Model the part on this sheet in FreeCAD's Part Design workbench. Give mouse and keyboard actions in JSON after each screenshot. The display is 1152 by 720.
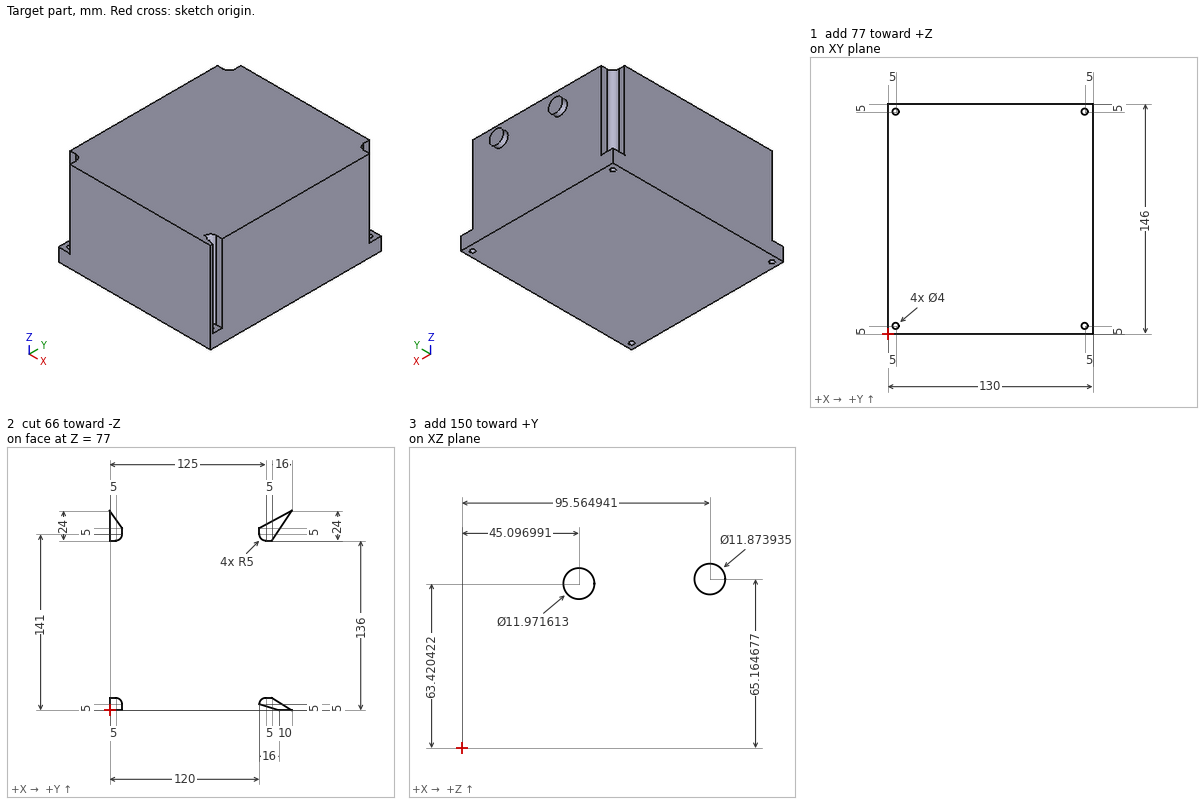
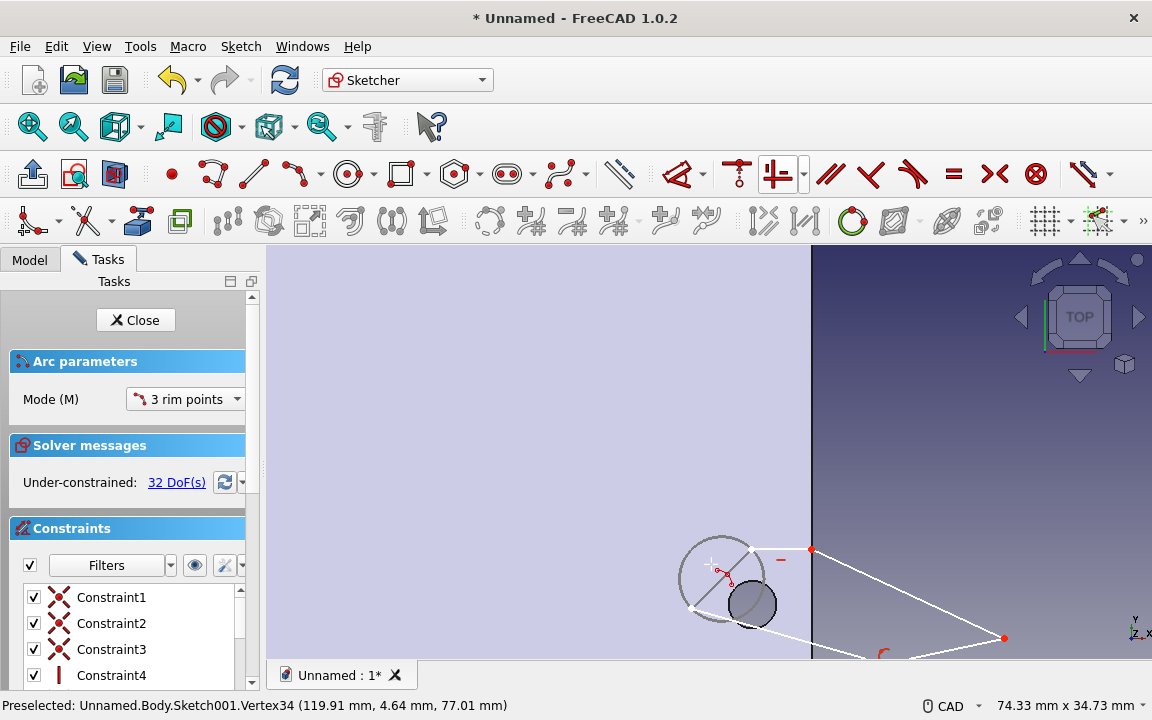
{"action": "left_click", "coordinate": [710, 562]}
{"action": "key", "text": "Escape"}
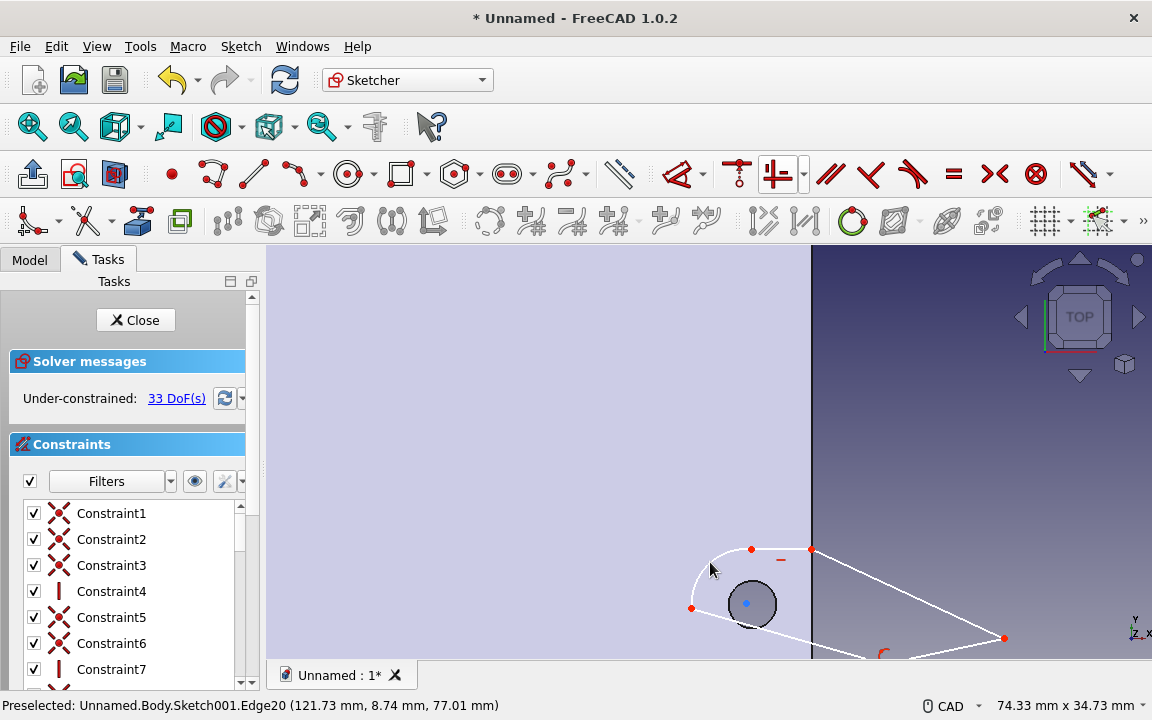
{"action": "scroll", "coordinate": [720, 568], "scroll_direction": "down", "scroll_amount": 10}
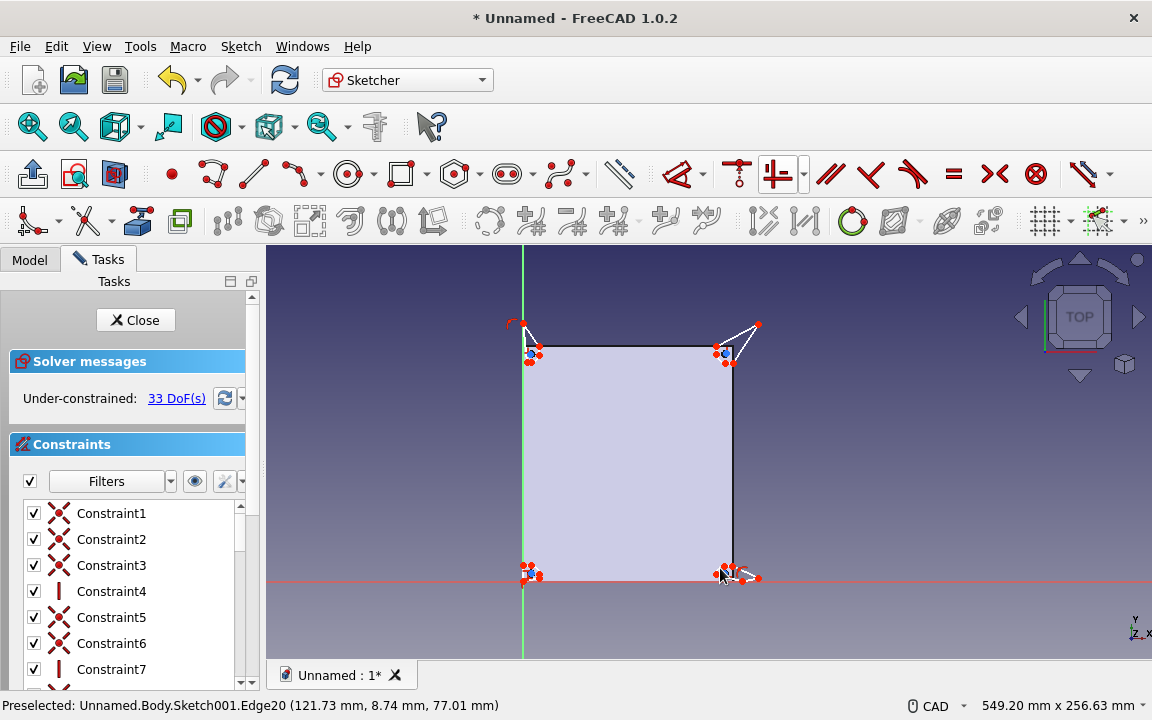
{"action": "scroll", "coordinate": [728, 363], "scroll_direction": "up", "scroll_amount": 9}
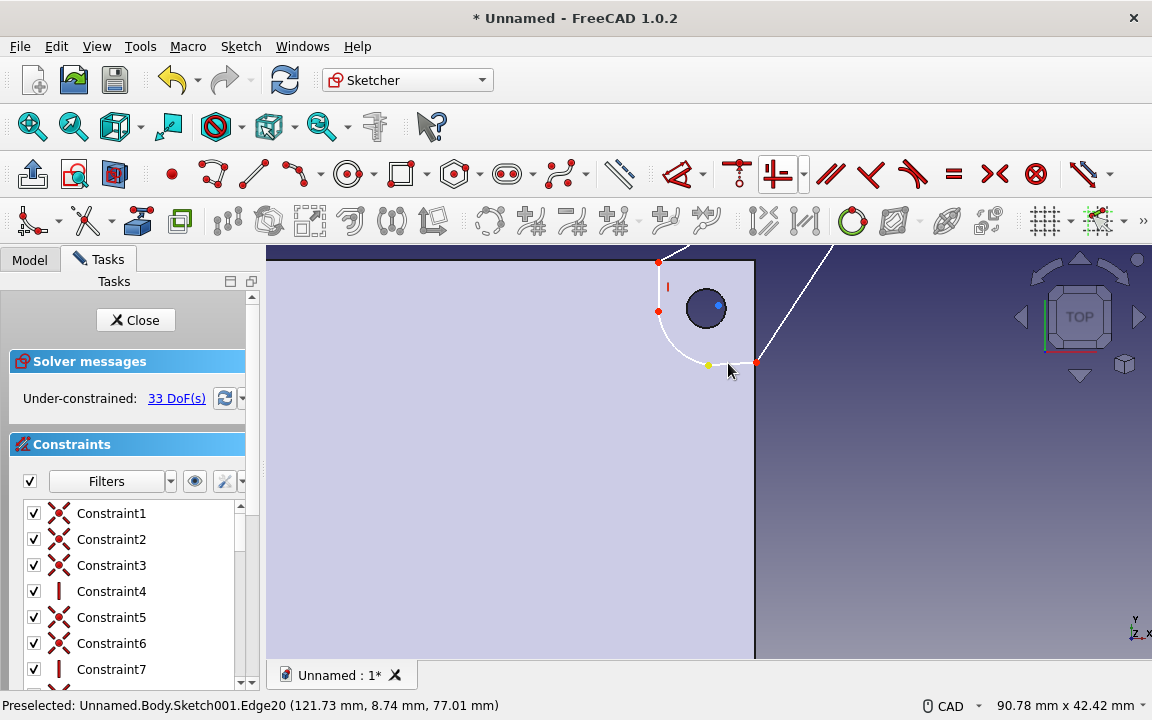
{"action": "left_click", "coordinate": [723, 364]}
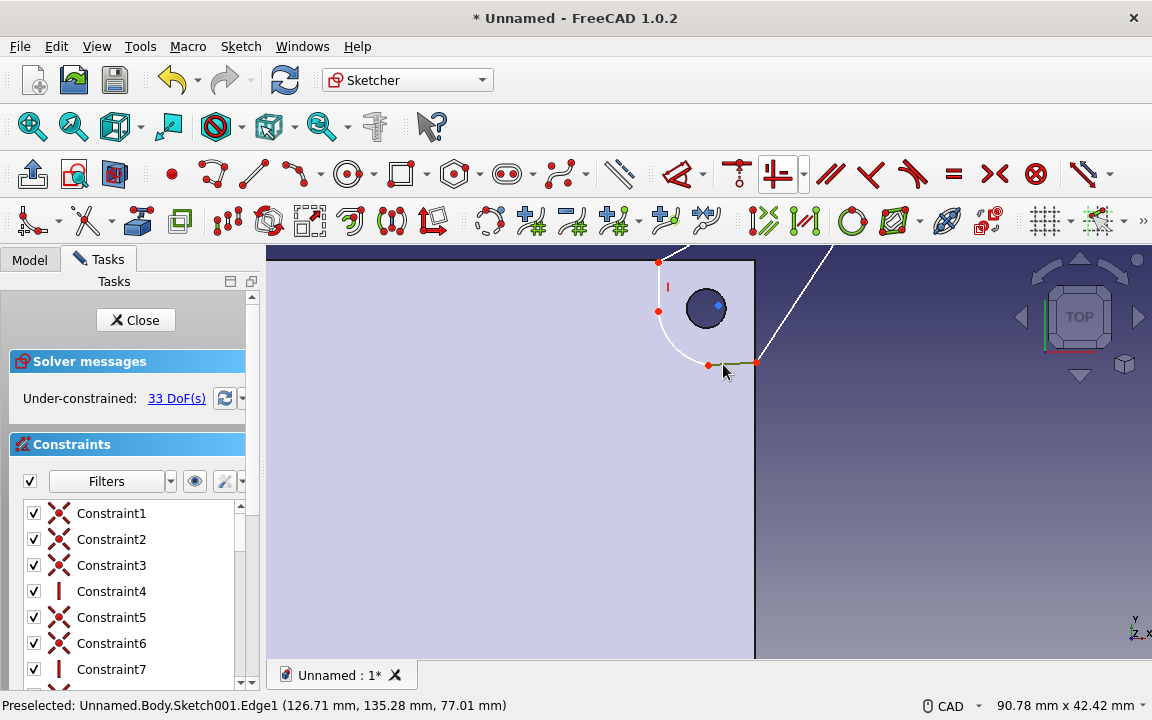
{"action": "left_click", "coordinate": [665, 334]}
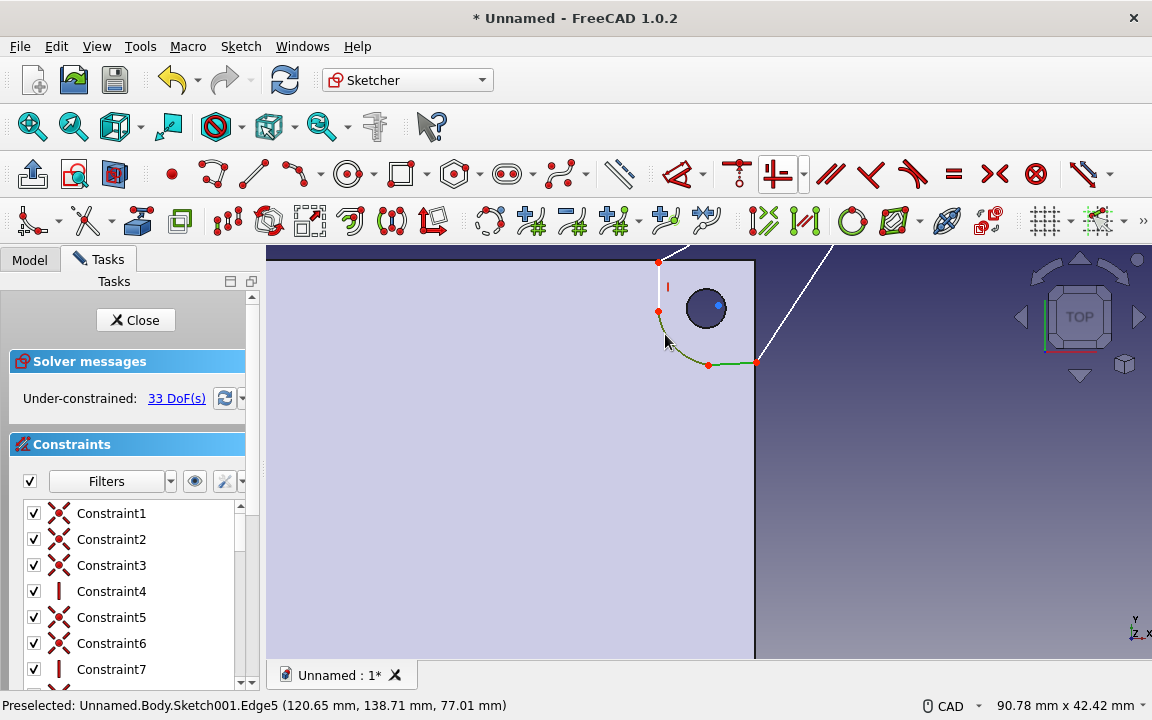
{"action": "left_click", "coordinate": [913, 174]}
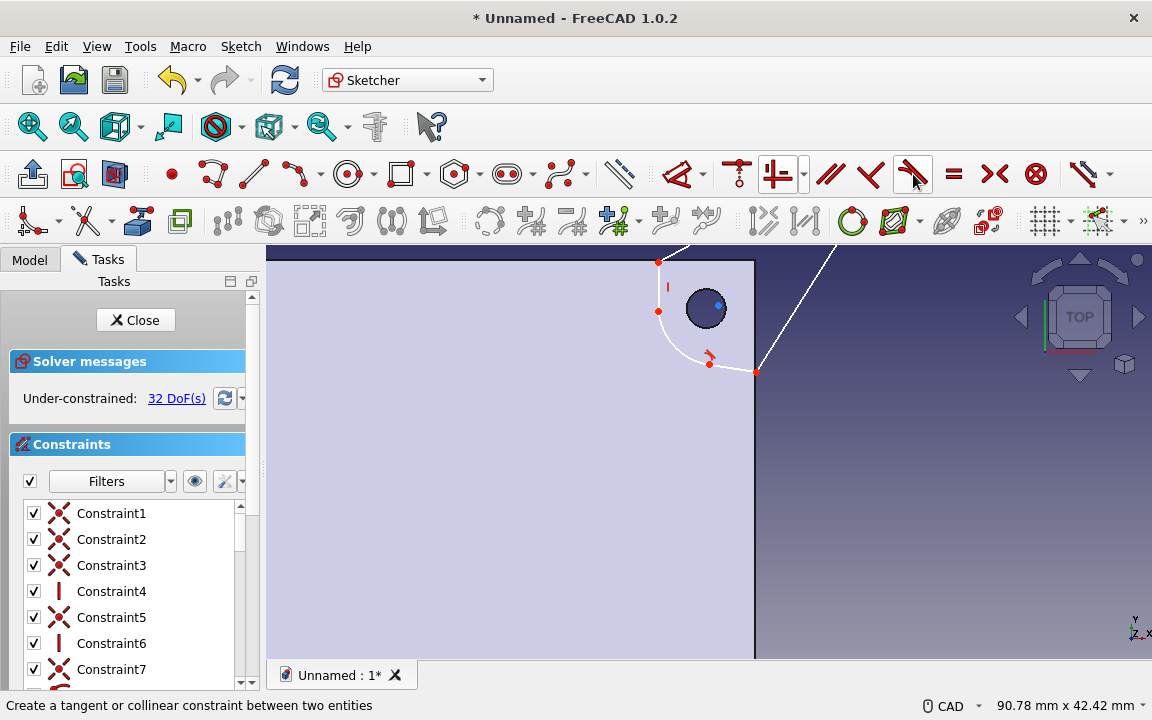
{"action": "left_click", "coordinate": [659, 277]}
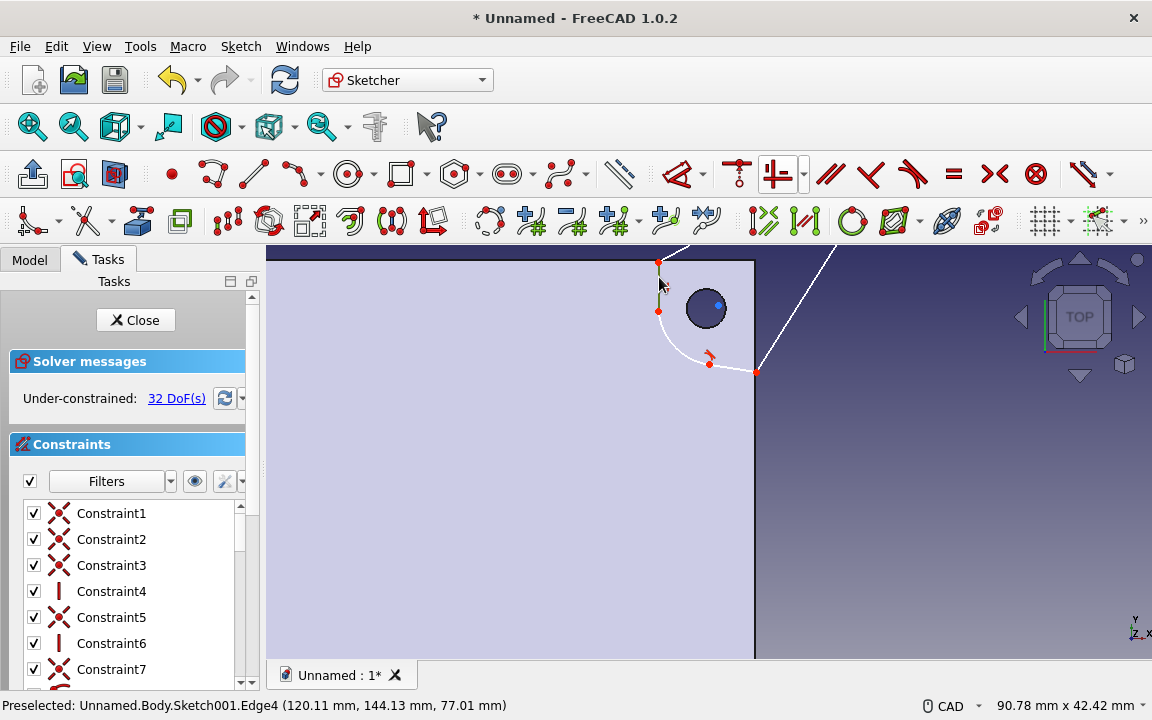
{"action": "left_click", "coordinate": [665, 334]}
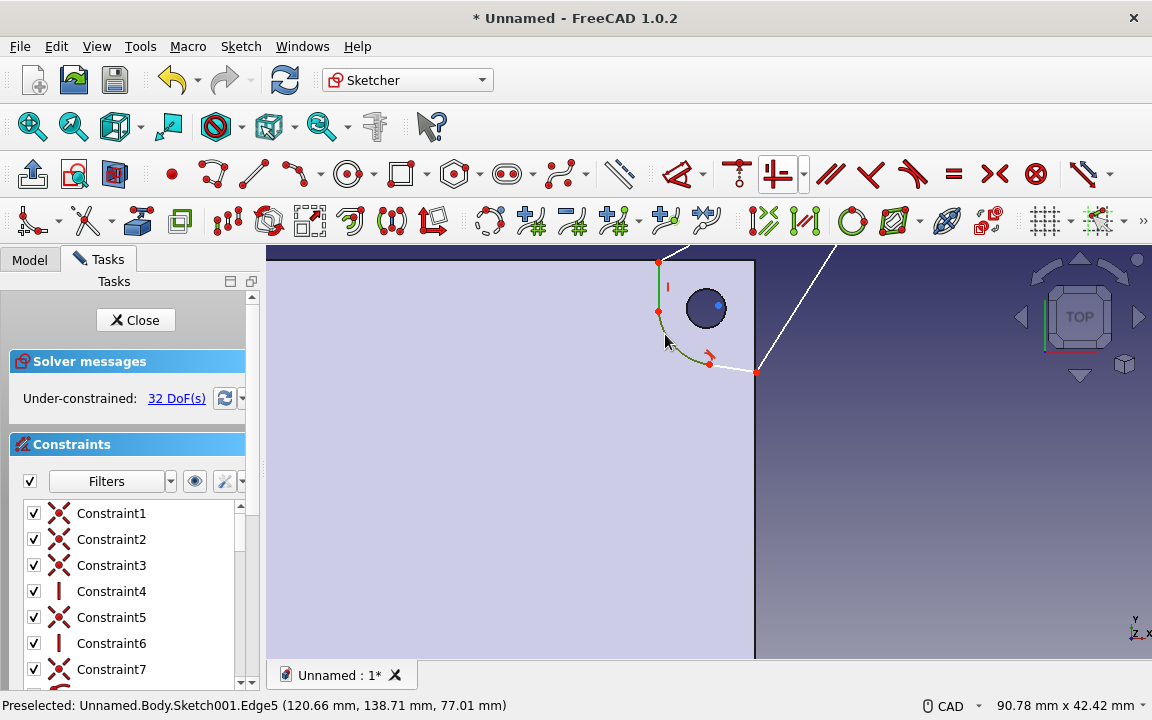
{"action": "left_click", "coordinate": [913, 174]}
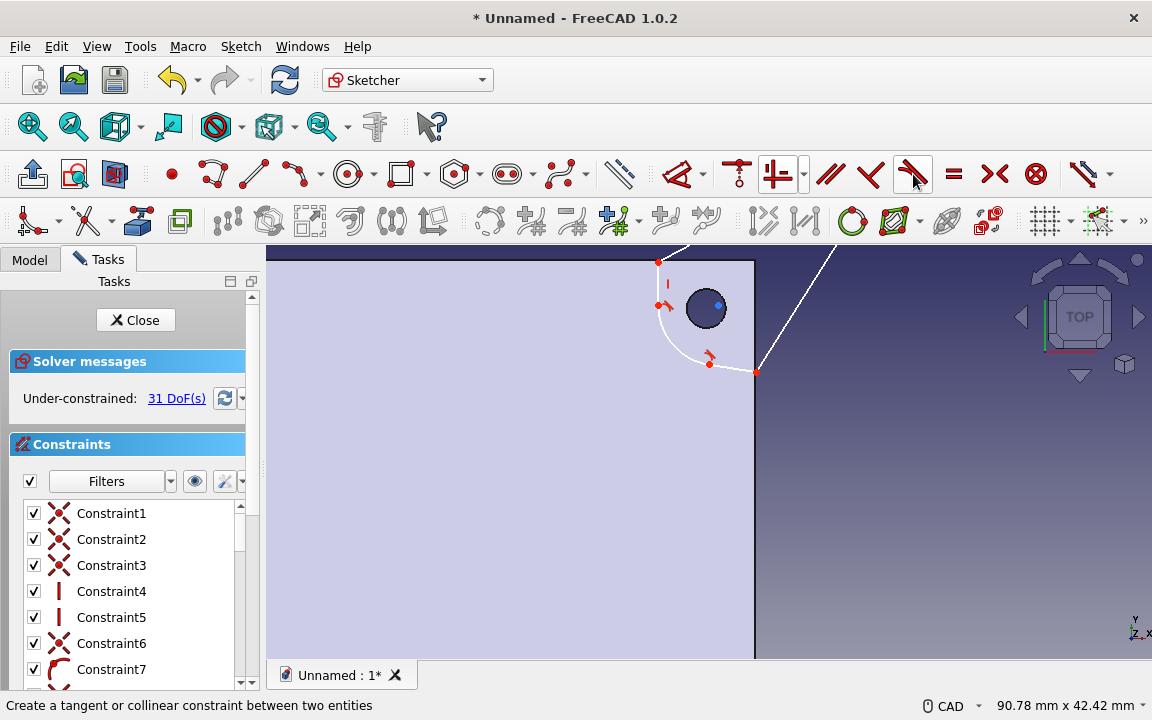
{"action": "scroll", "coordinate": [728, 363], "scroll_direction": "down", "scroll_amount": 9}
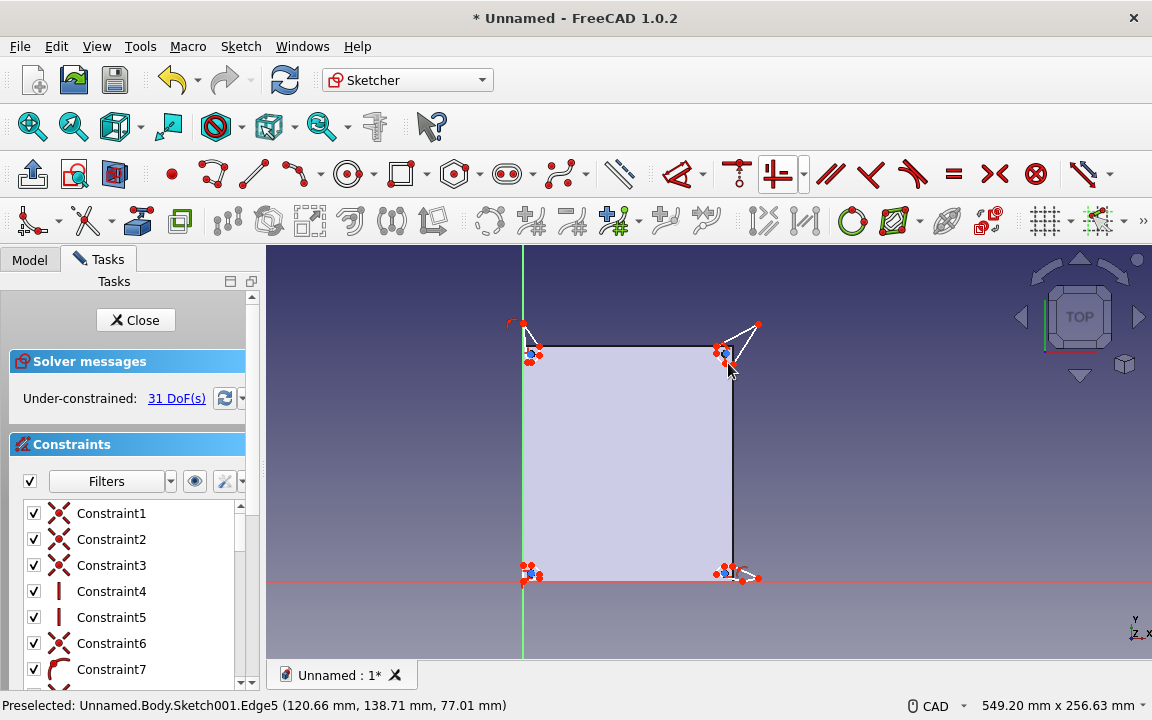
{"action": "scroll", "coordinate": [539, 353], "scroll_direction": "up", "scroll_amount": 9}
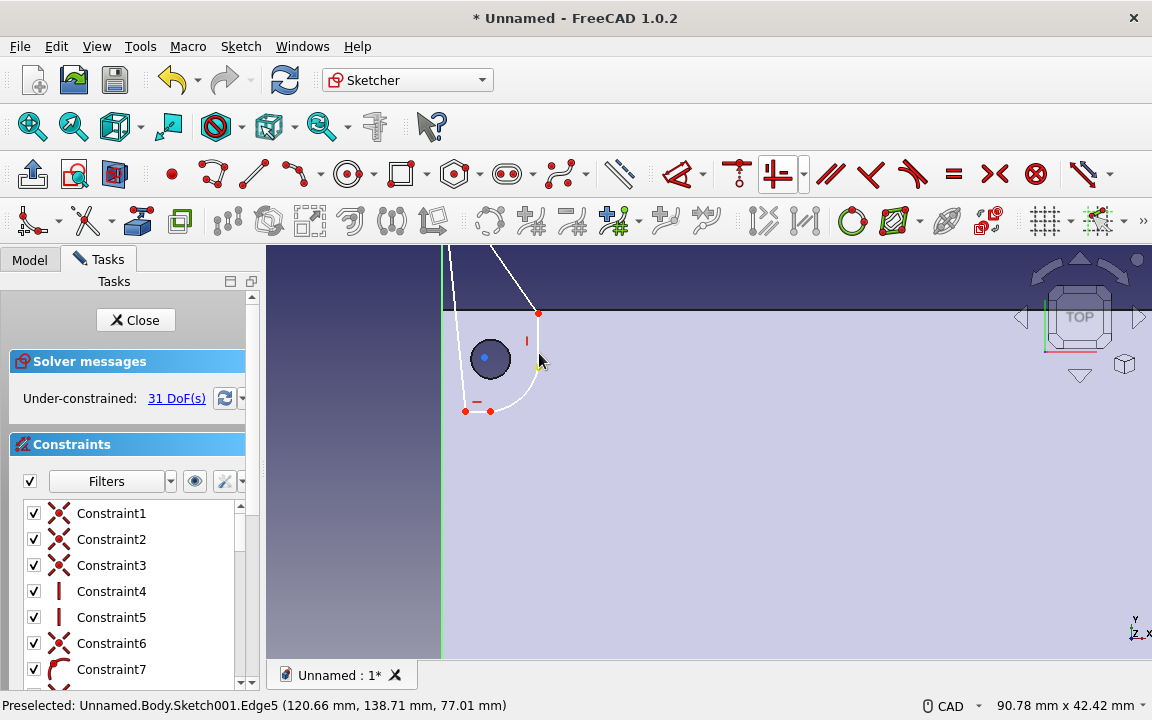
{"action": "left_click", "coordinate": [538, 351]}